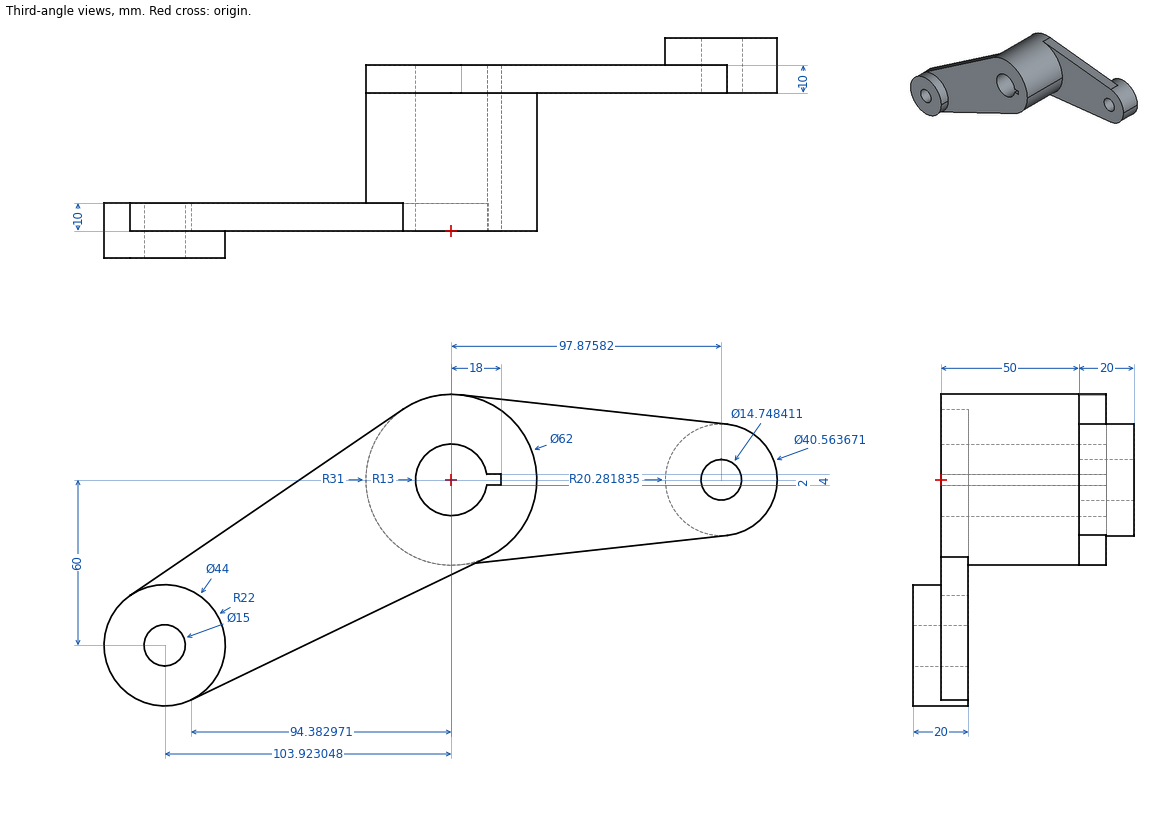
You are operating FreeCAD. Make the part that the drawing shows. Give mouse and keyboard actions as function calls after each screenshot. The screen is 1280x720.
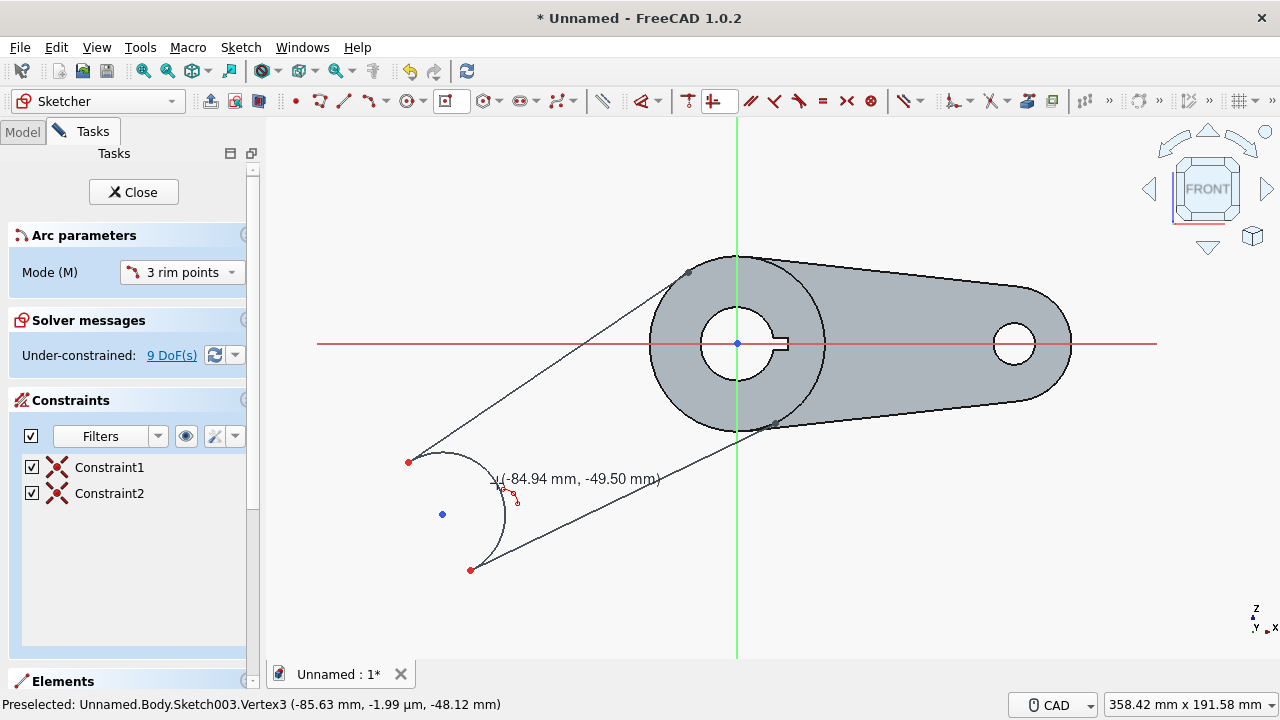
click(775, 424)
click(688, 273)
click(661, 388)
key(Escape)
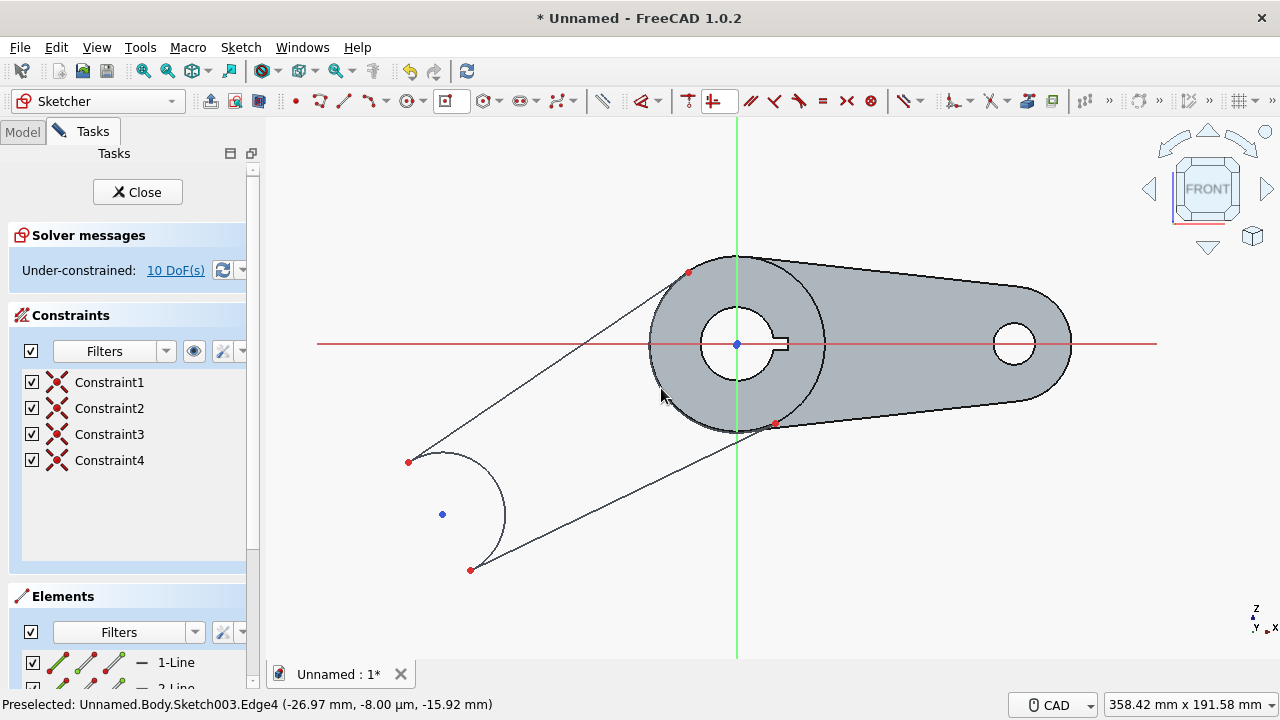
click(604, 330)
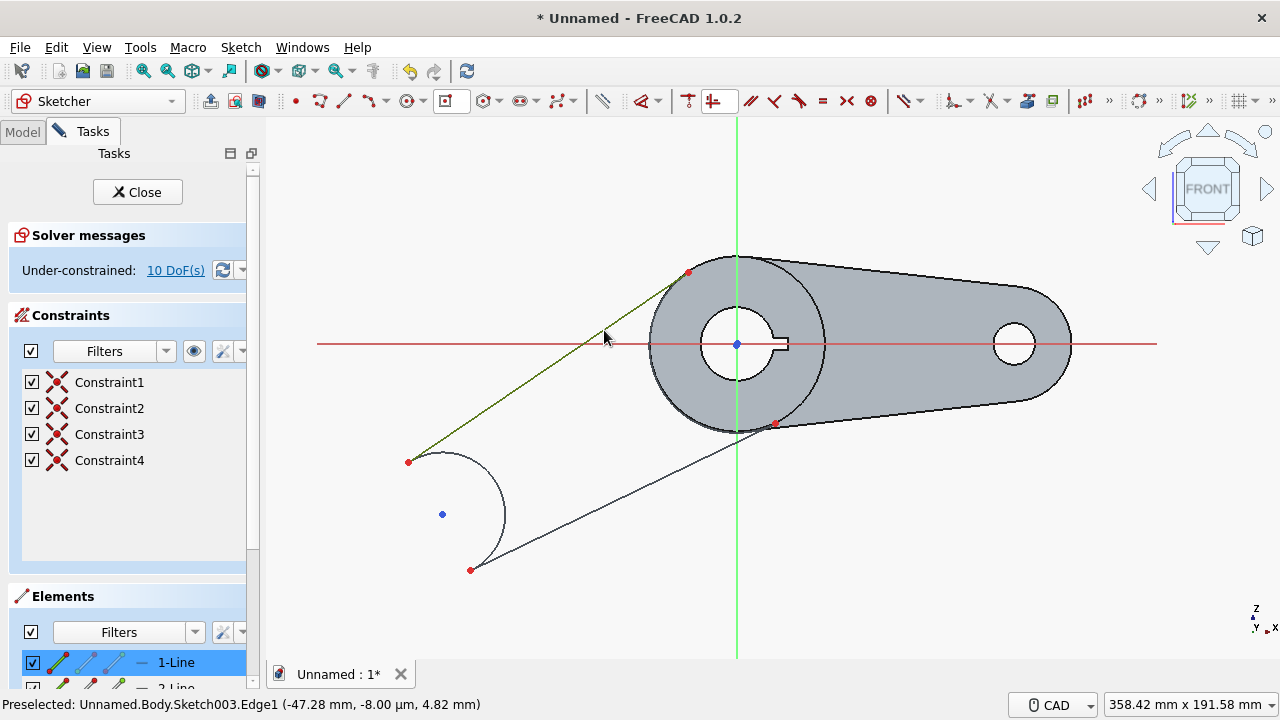
click(505, 523)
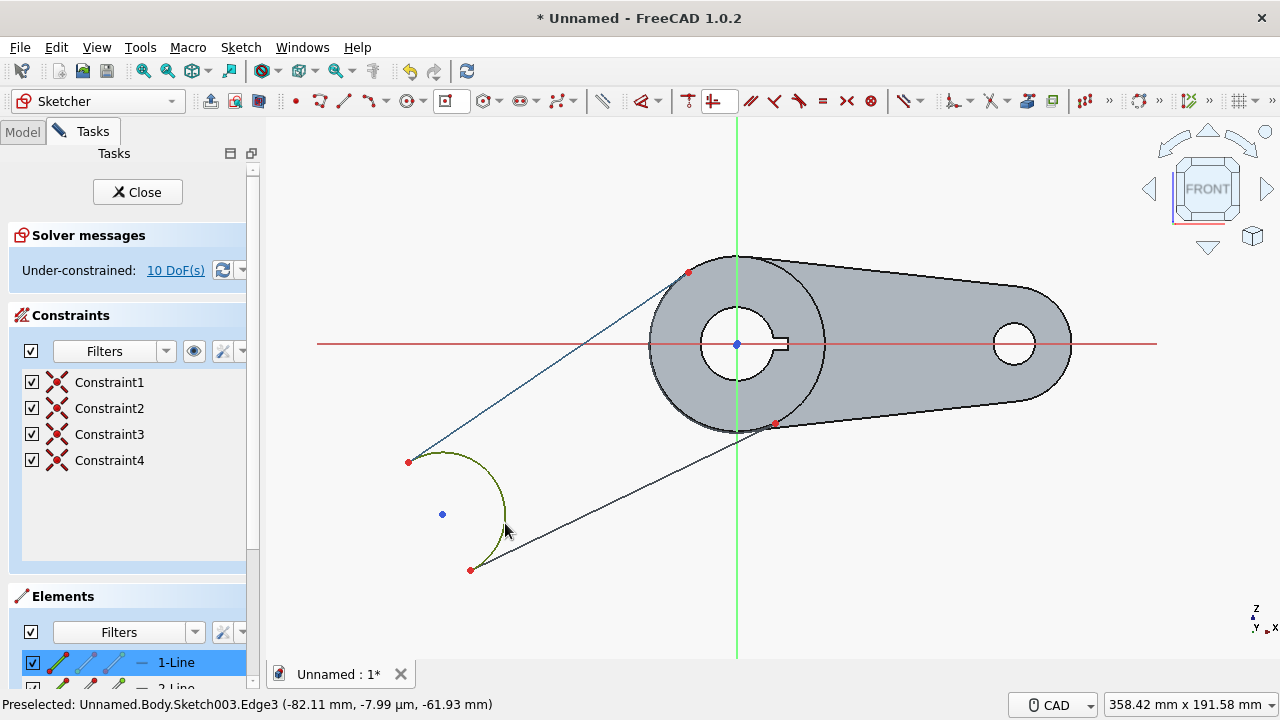
click(800, 102)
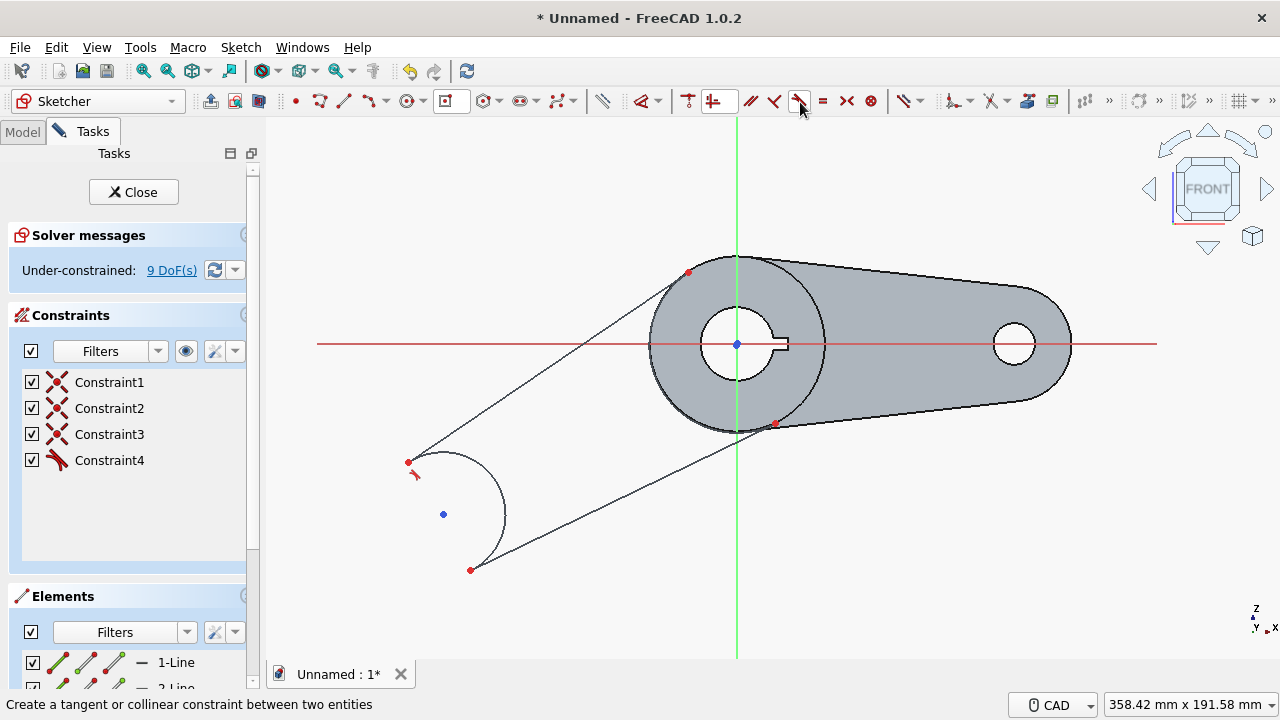
click(604, 330)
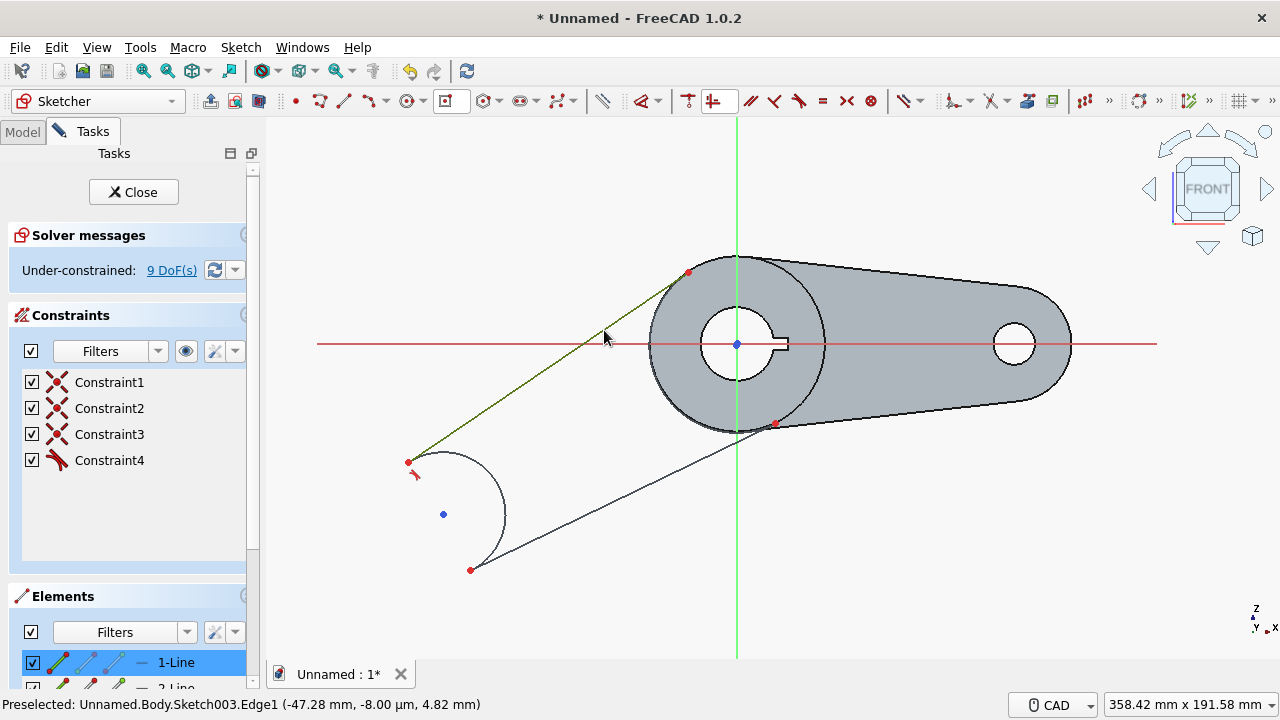
click(699, 424)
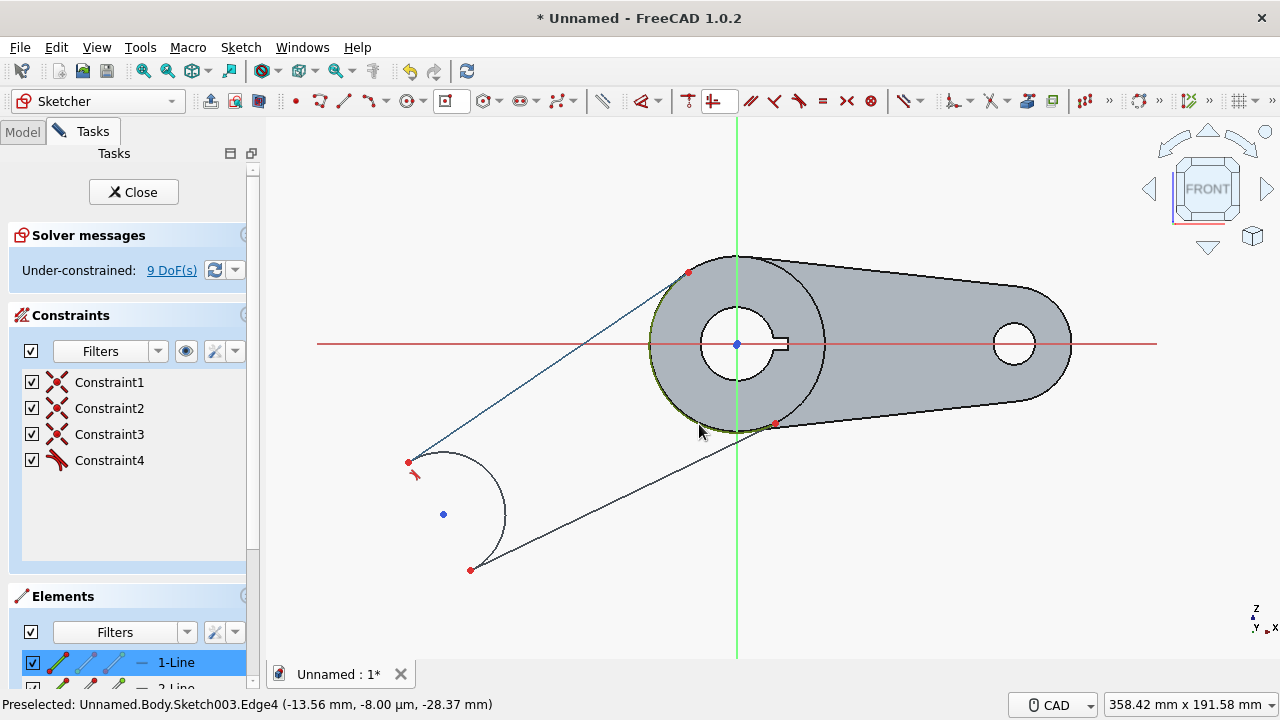
click(800, 102)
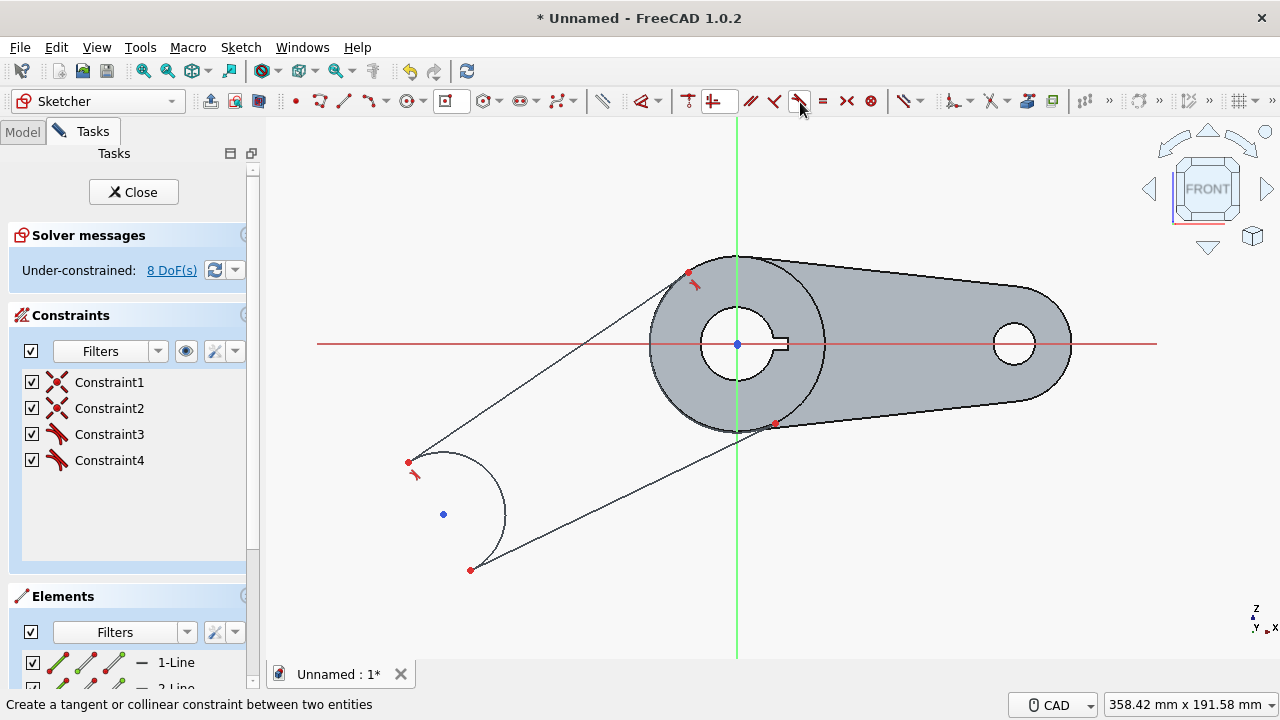
click(562, 527)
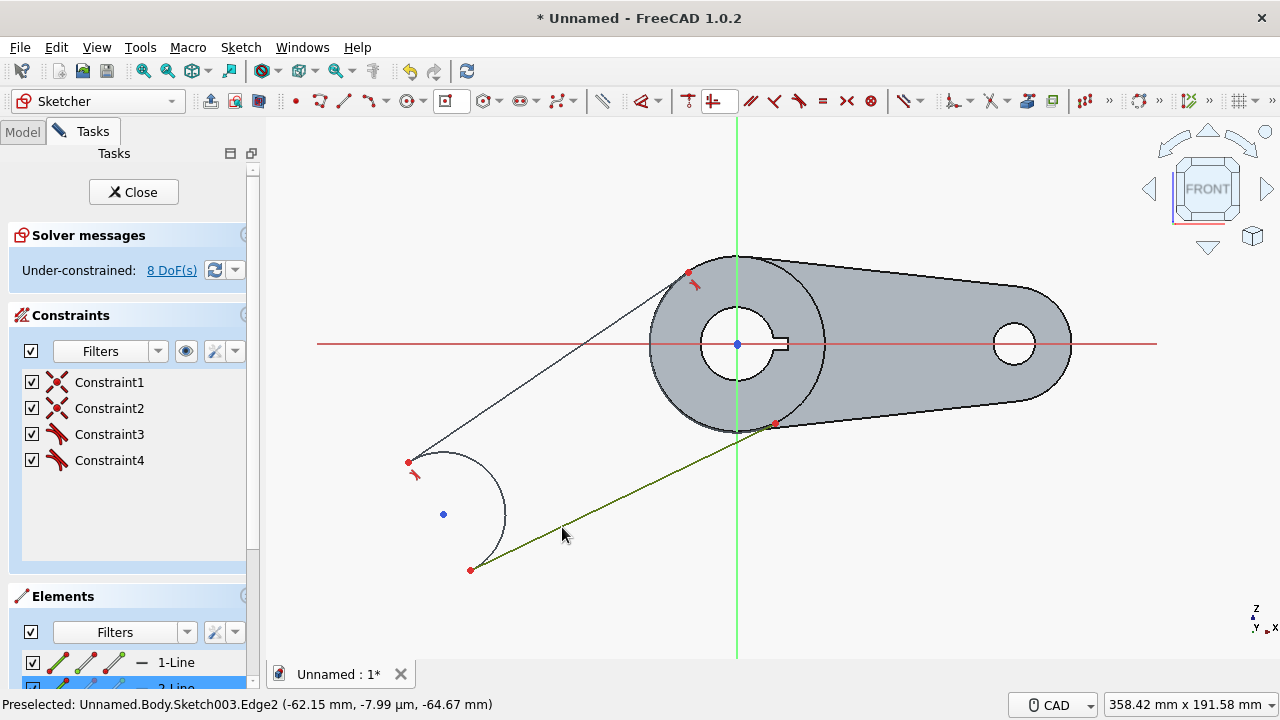
click(505, 523)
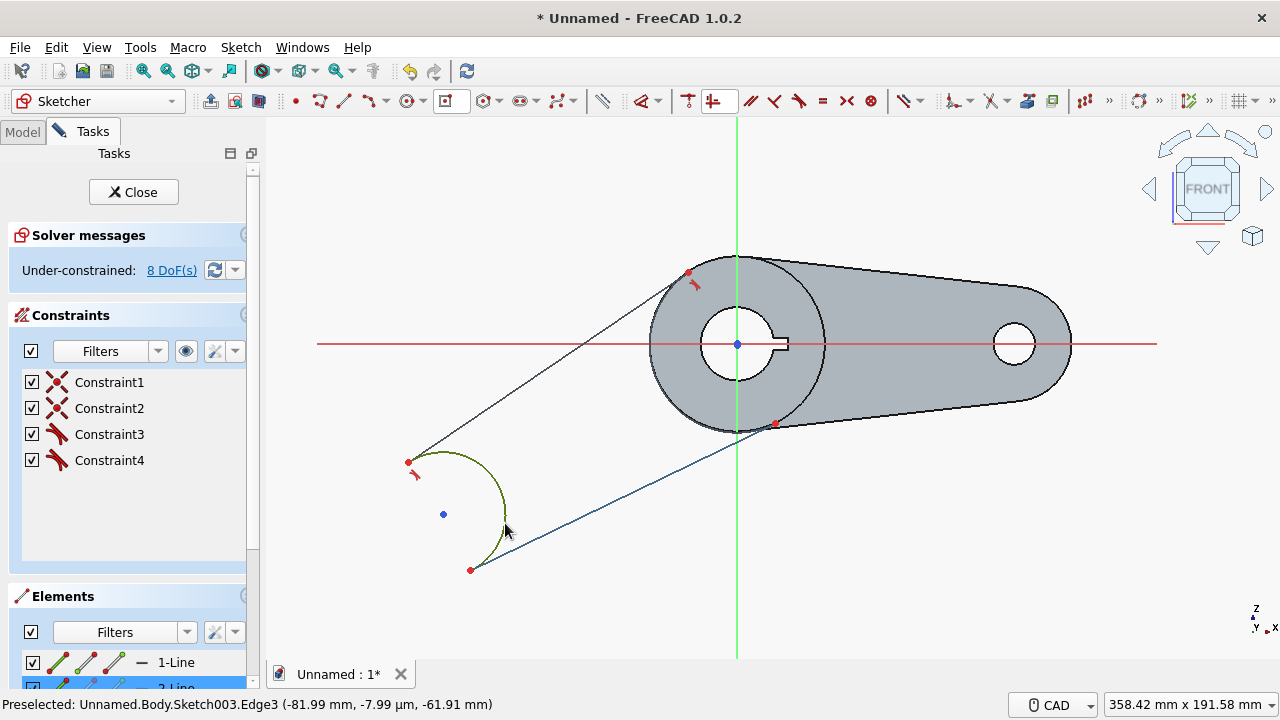
key(t)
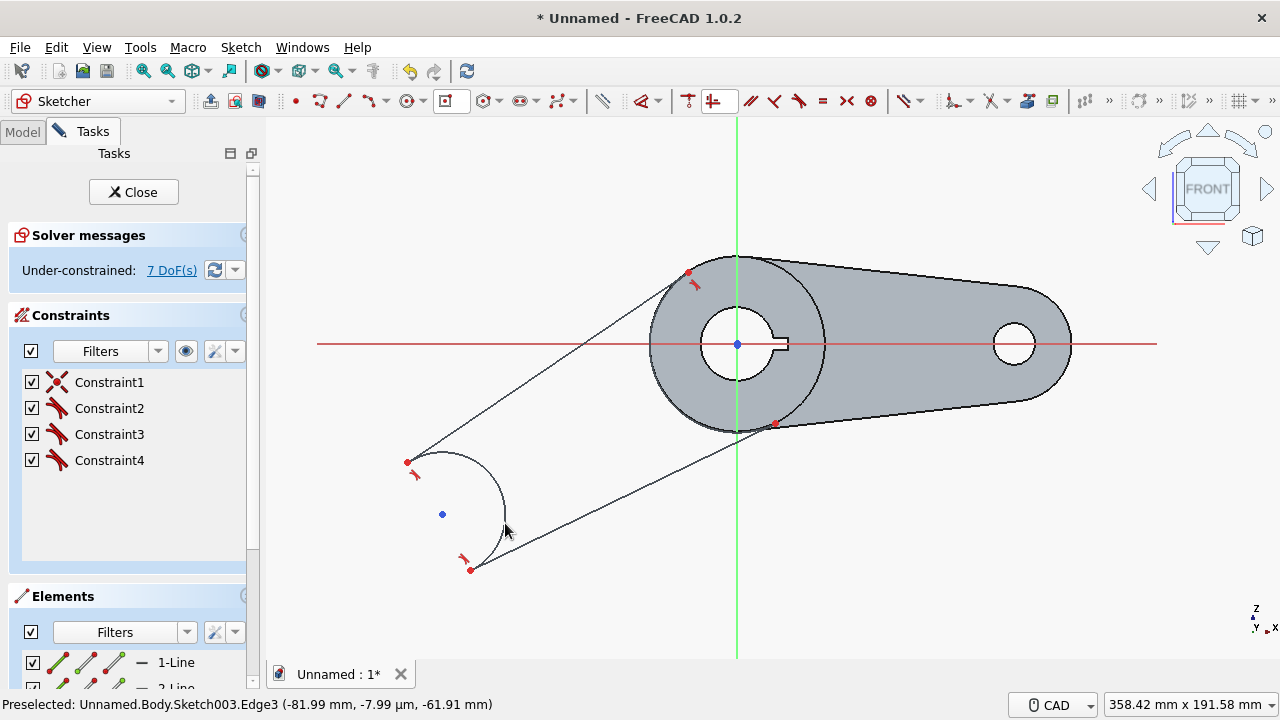
click(562, 527)